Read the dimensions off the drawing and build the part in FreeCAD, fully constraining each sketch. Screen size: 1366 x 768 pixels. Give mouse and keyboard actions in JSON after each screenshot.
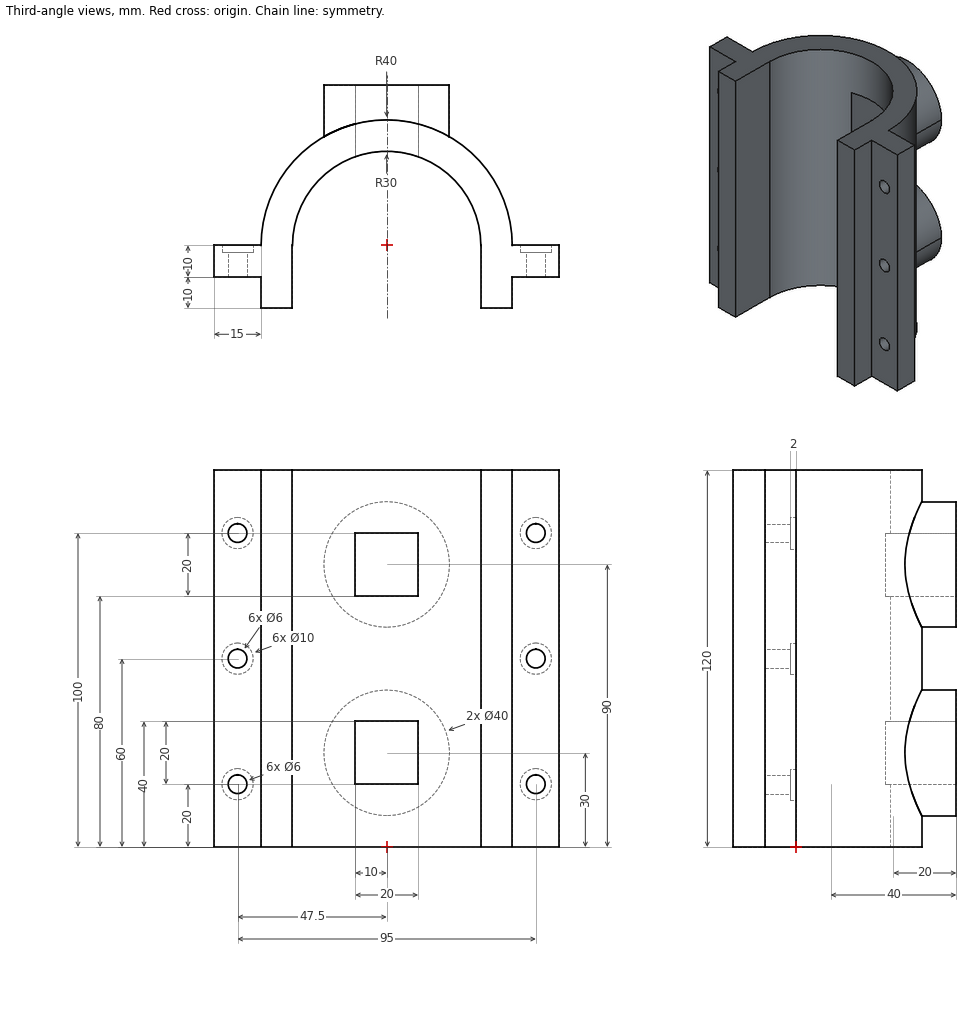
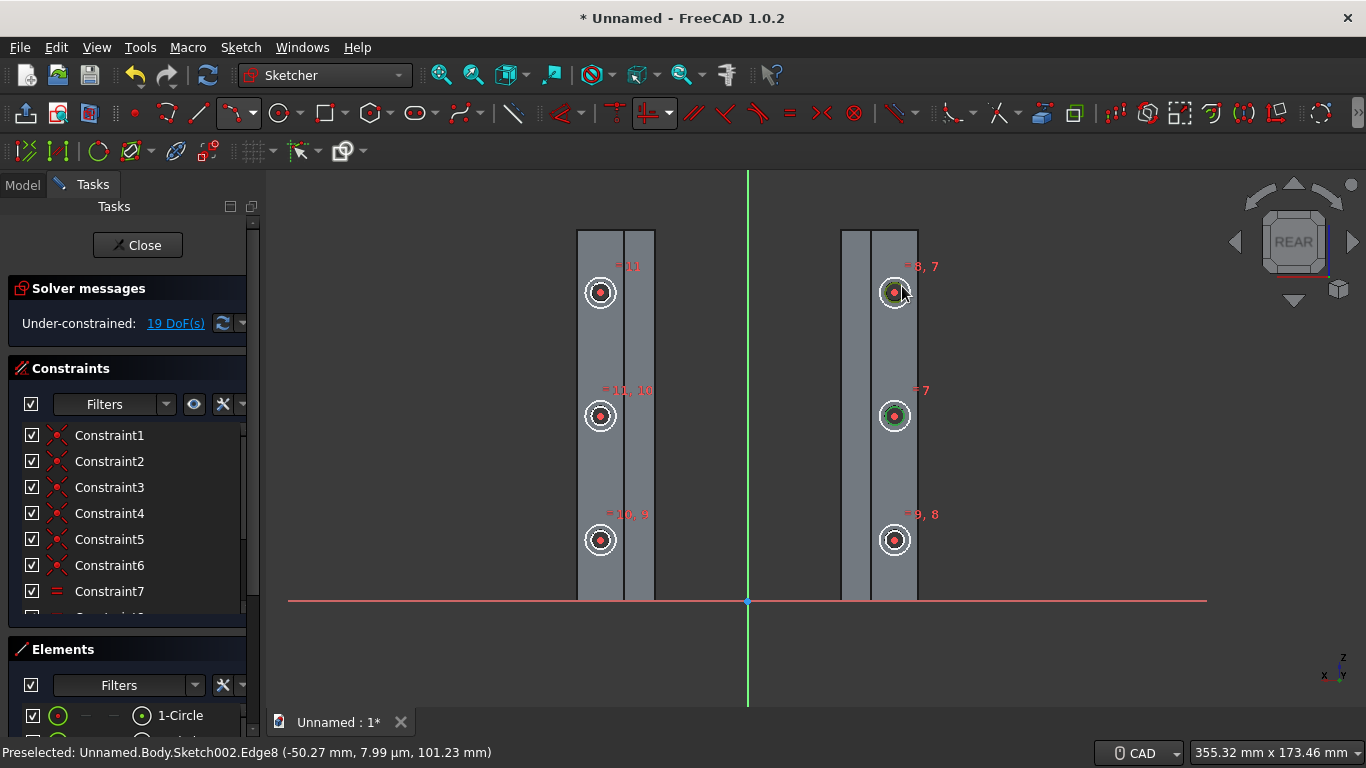
{"action": "scroll", "coordinate": [901, 534], "scroll_direction": "up", "scroll_amount": 5}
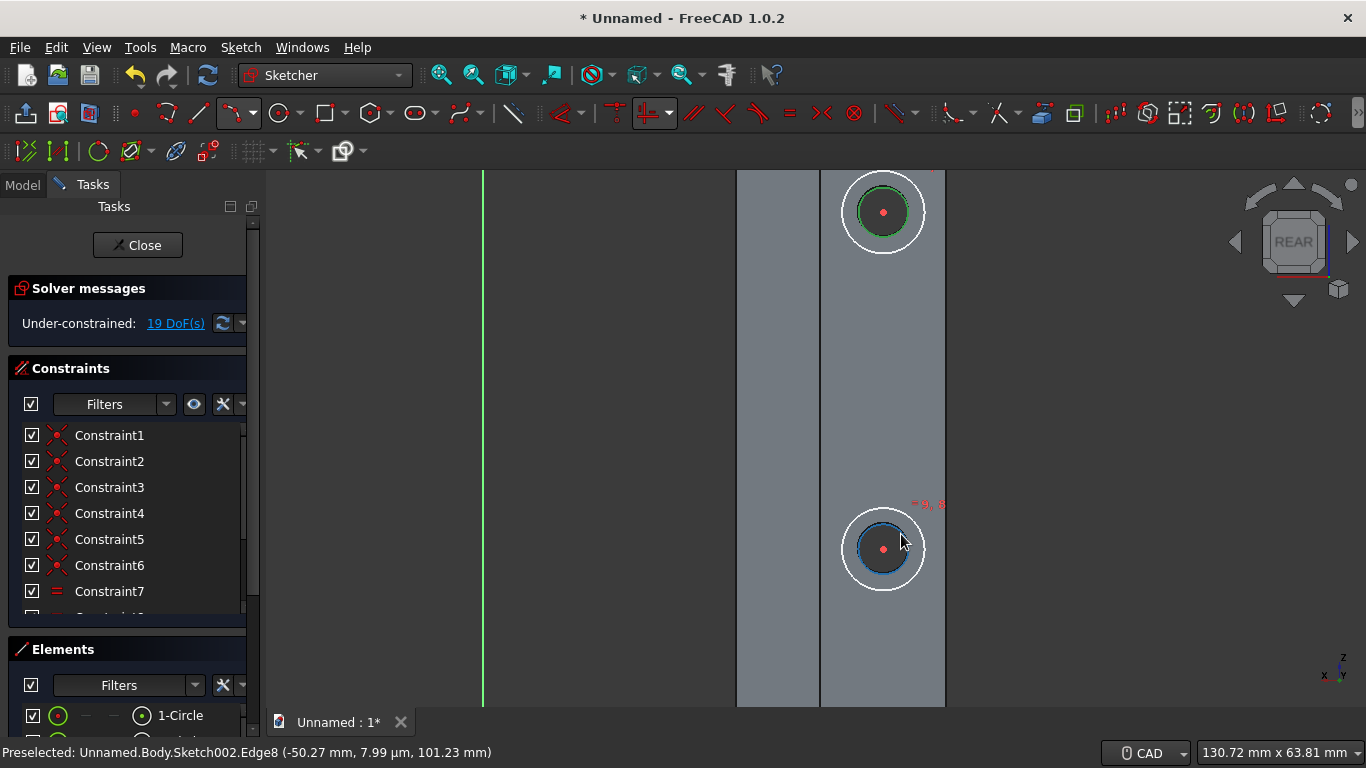
{"action": "left_click", "coordinate": [901, 532]}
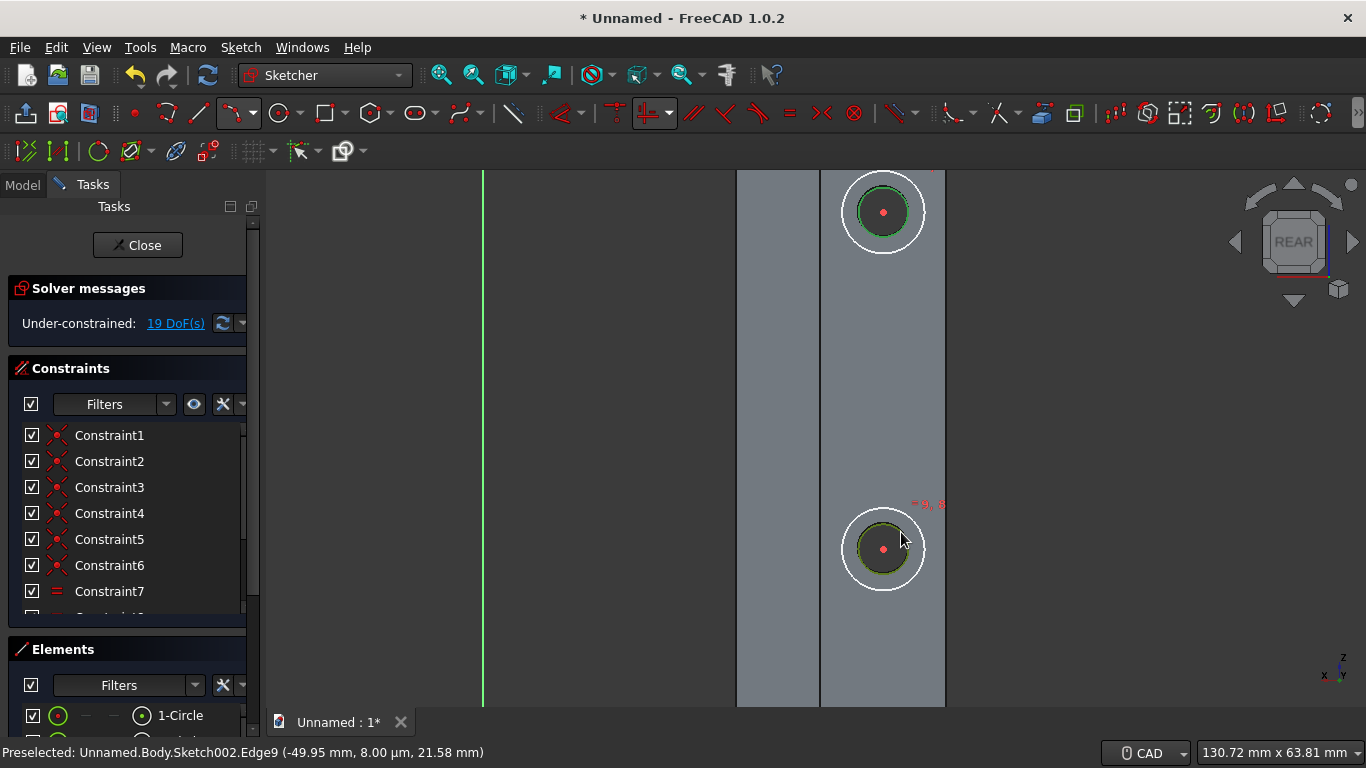
{"action": "scroll", "coordinate": [901, 534], "scroll_direction": "down", "scroll_amount": 5}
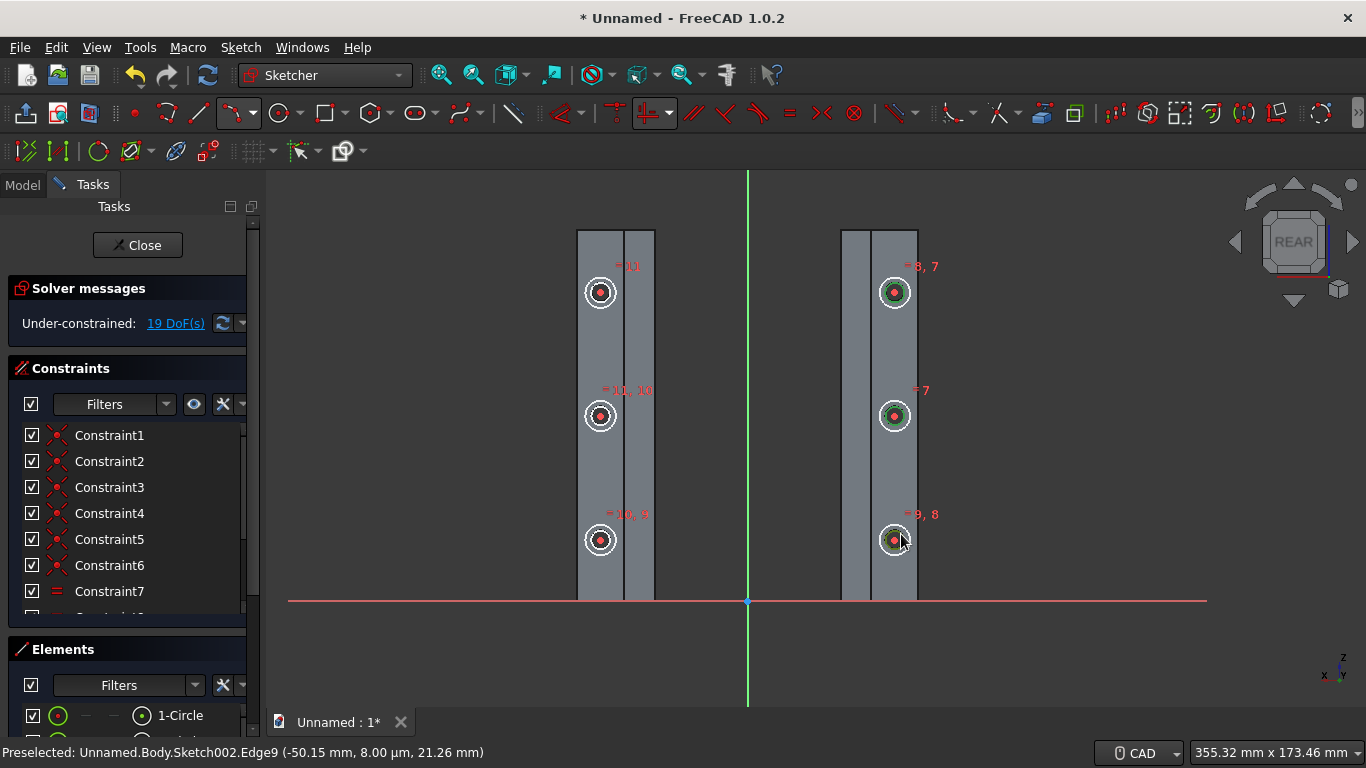
{"action": "scroll", "coordinate": [607, 533], "scroll_direction": "up", "scroll_amount": 5}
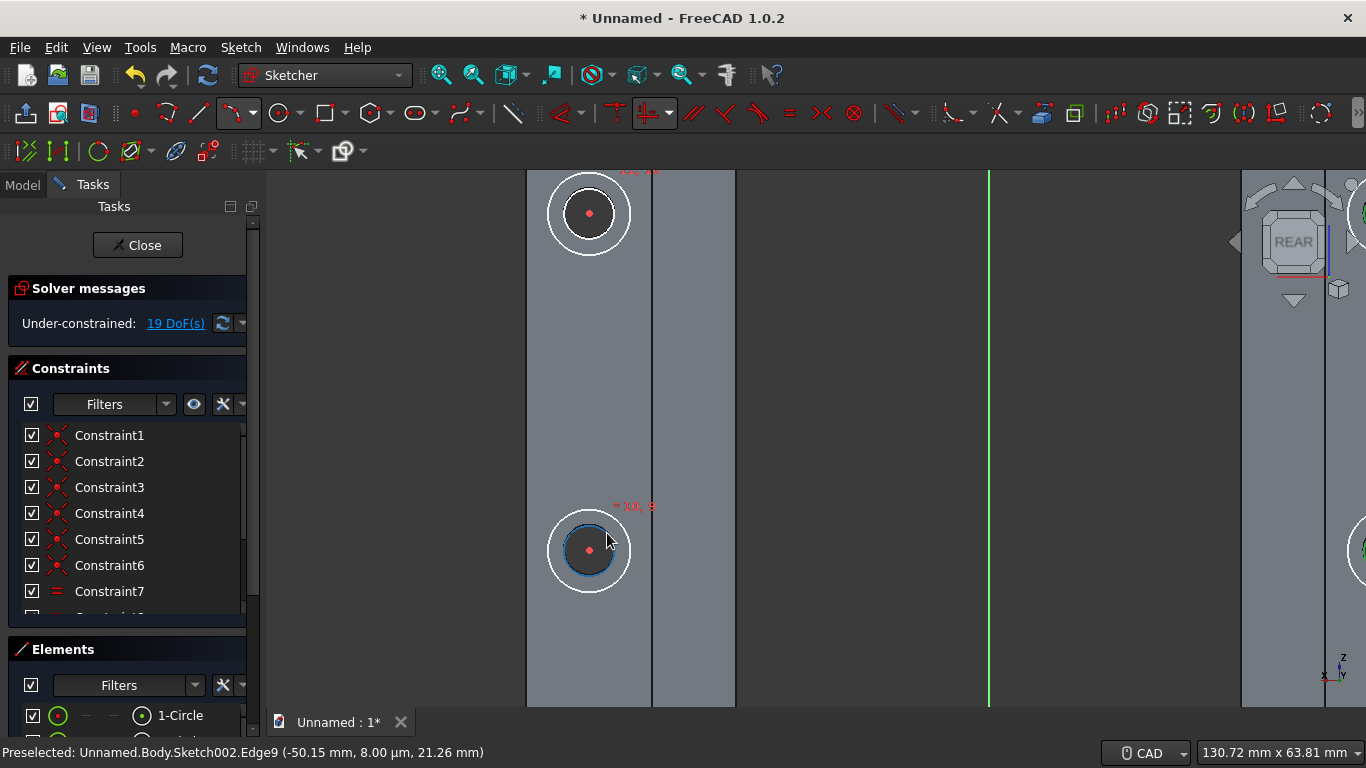
{"action": "left_click", "coordinate": [607, 533]}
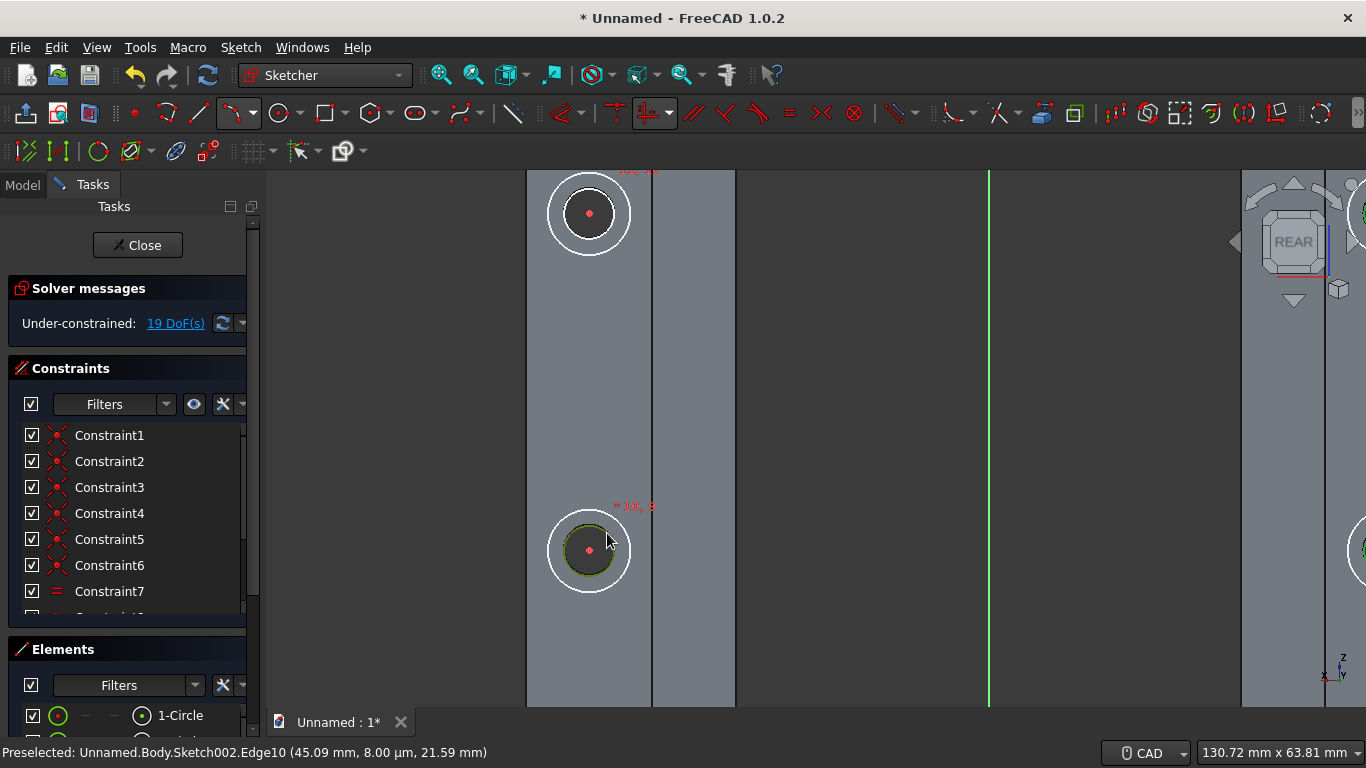
{"action": "left_click", "coordinate": [572, 232]}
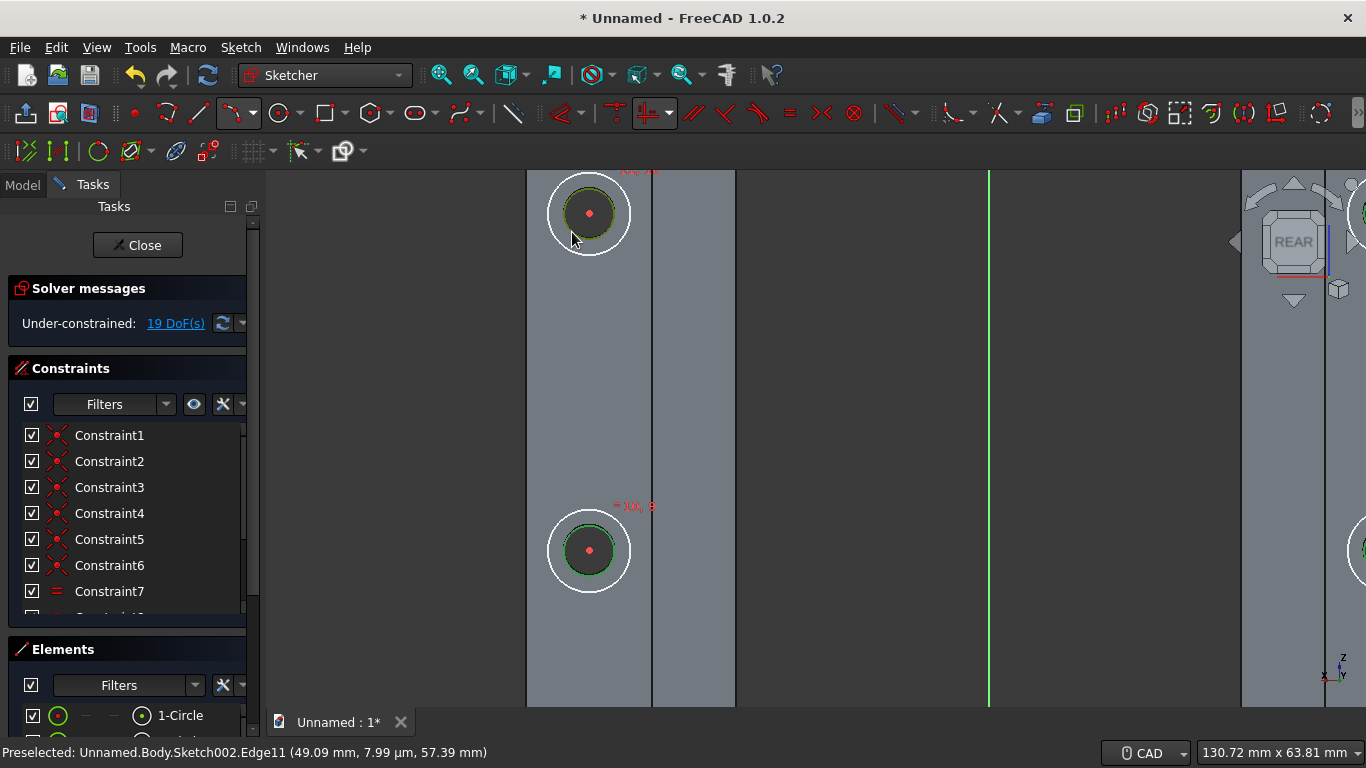
{"action": "scroll", "coordinate": [607, 533], "scroll_direction": "down", "scroll_amount": 5}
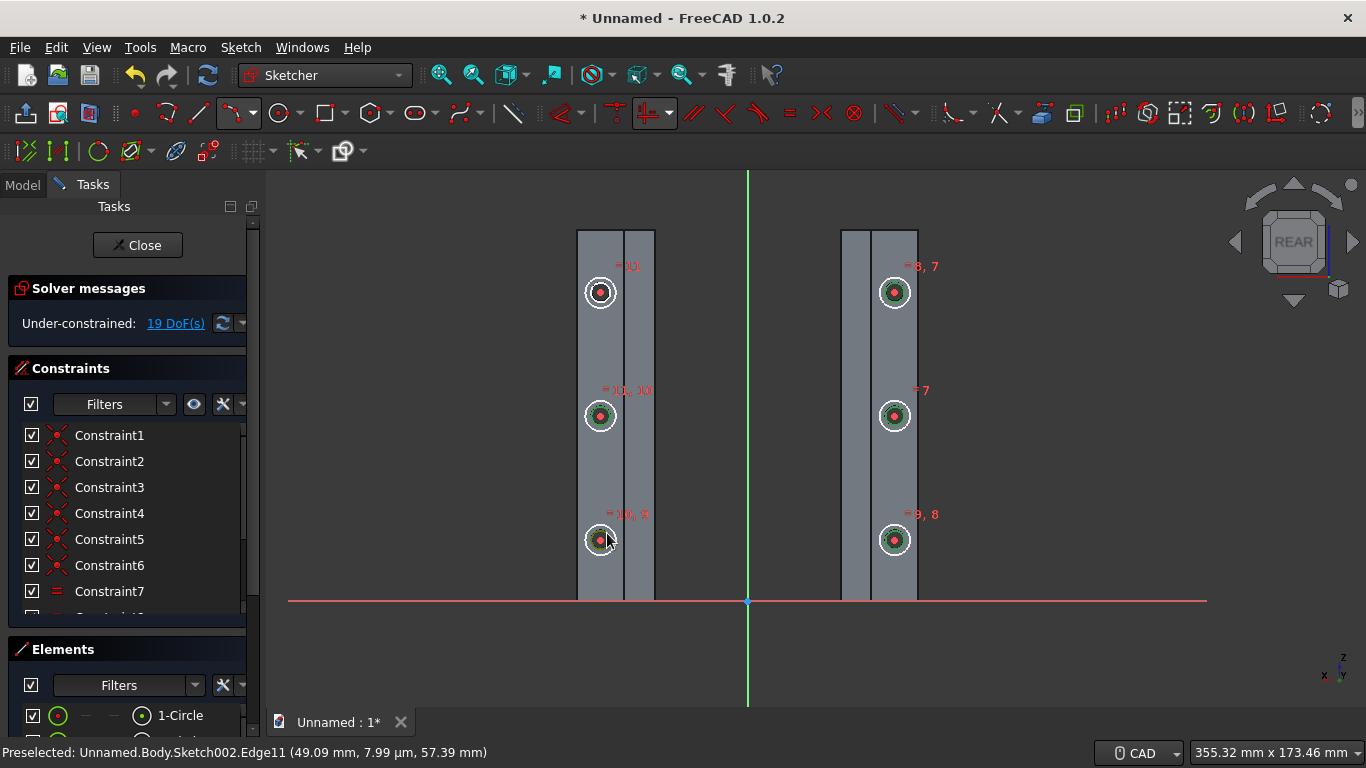
{"action": "scroll", "coordinate": [607, 286], "scroll_direction": "up", "scroll_amount": 5}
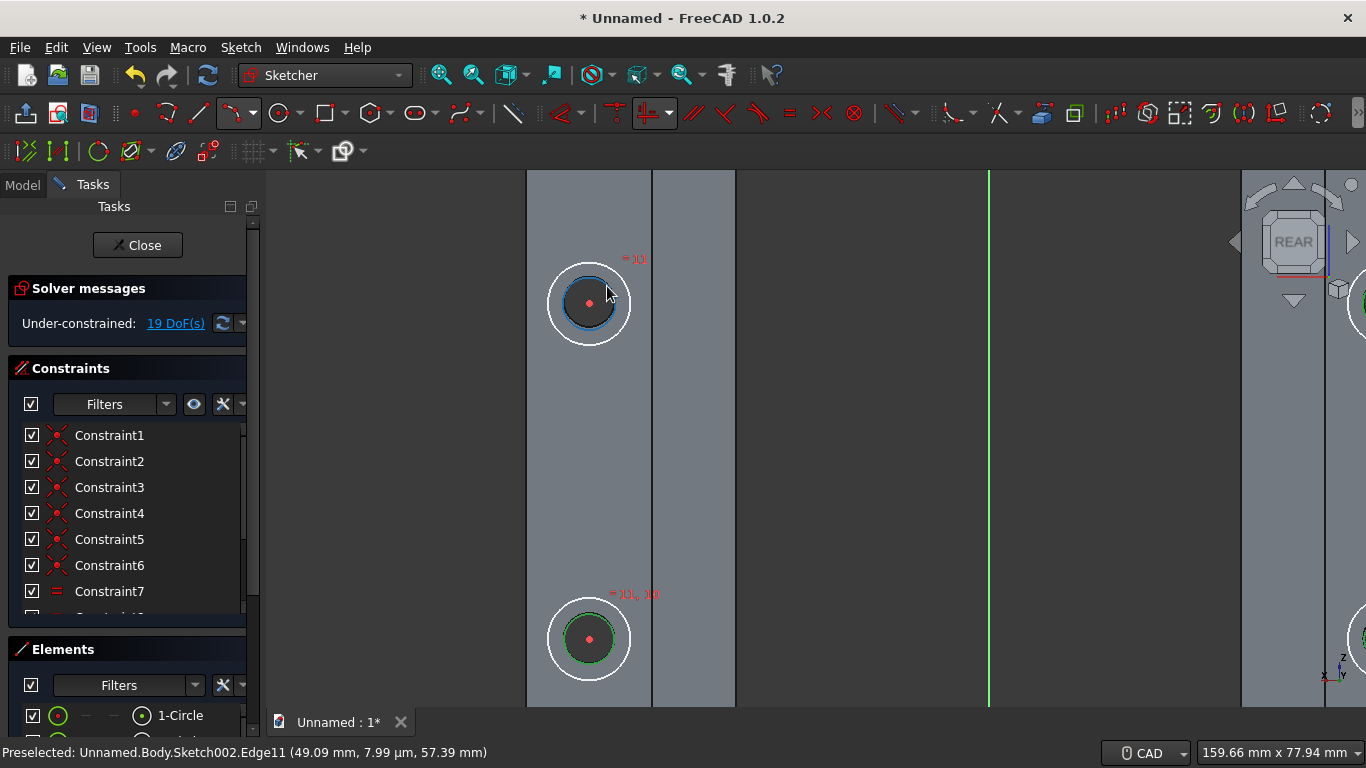
{"action": "left_click", "coordinate": [608, 285]}